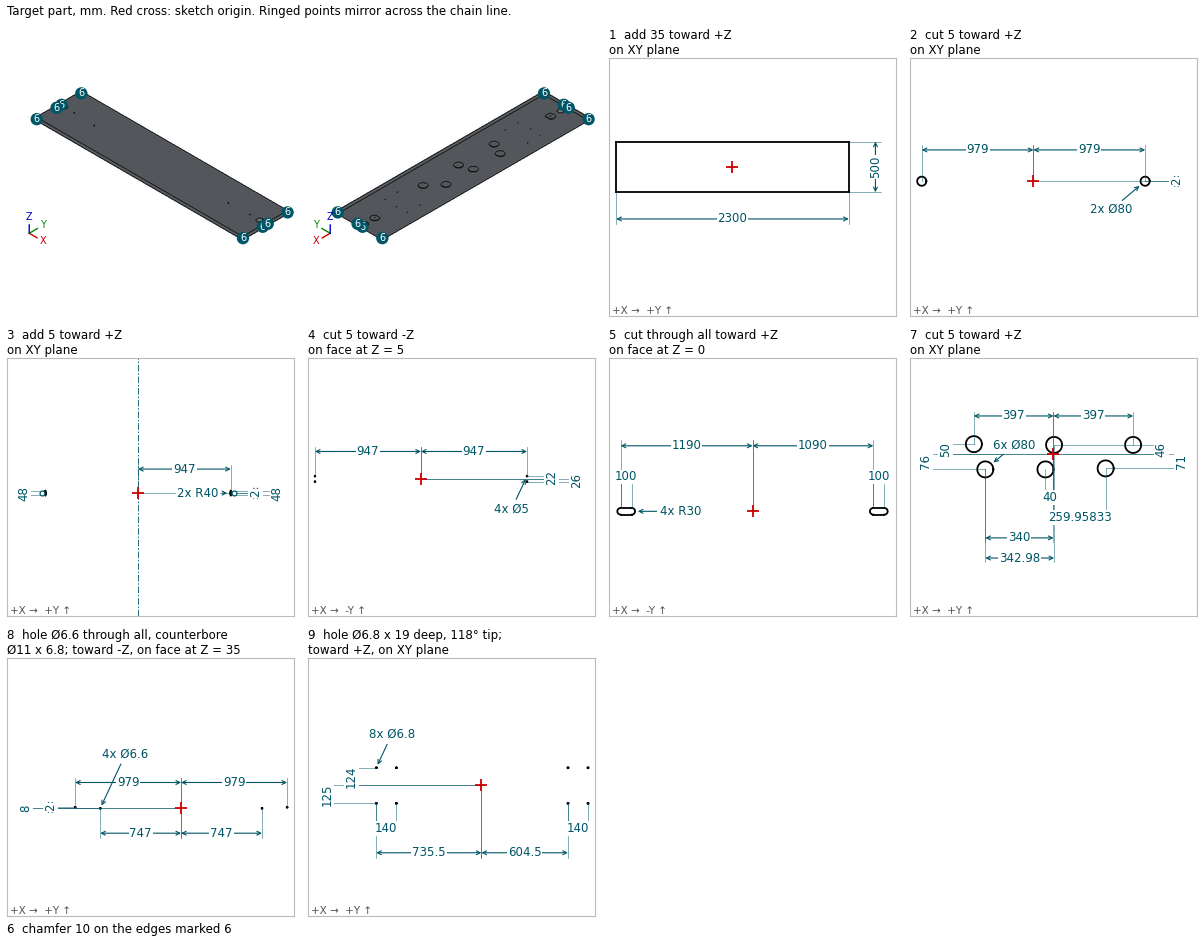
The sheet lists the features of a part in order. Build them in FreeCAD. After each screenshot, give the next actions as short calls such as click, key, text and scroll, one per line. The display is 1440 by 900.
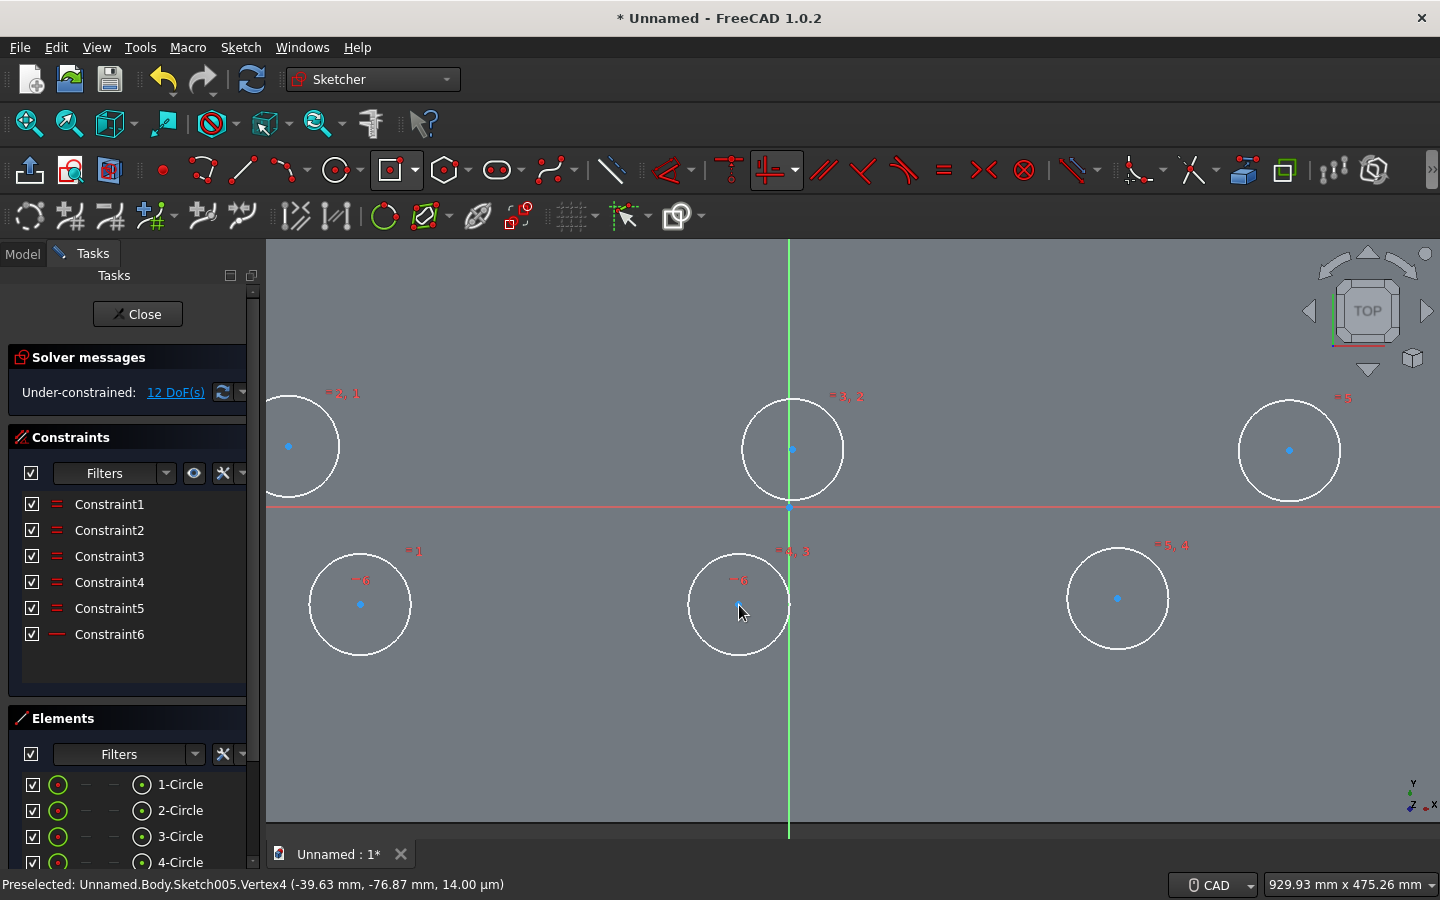
click(793, 450)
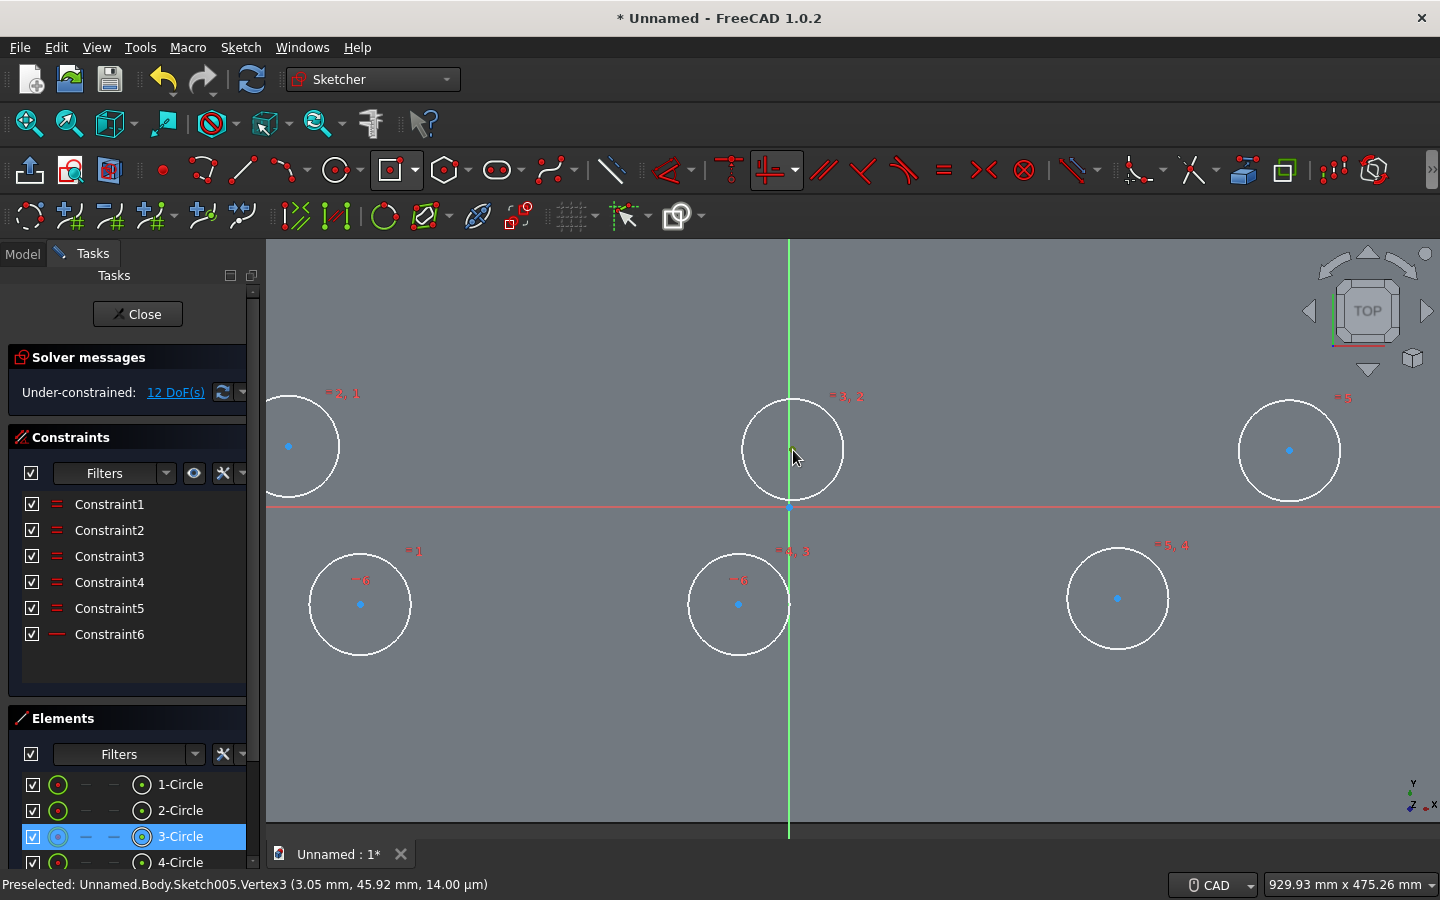
scroll(775, 570, down, 2)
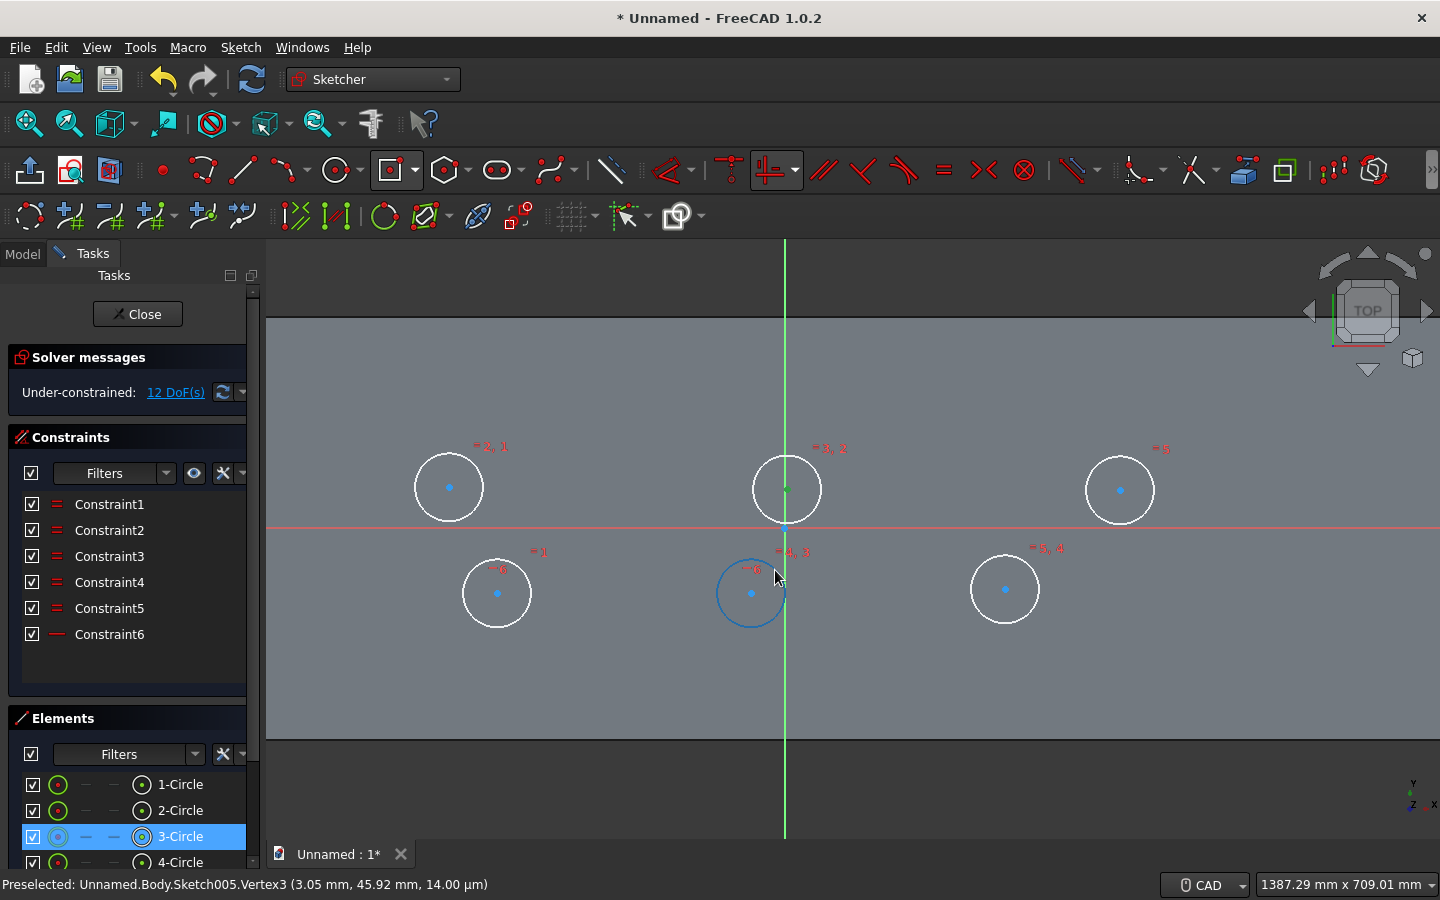
click(1120, 490)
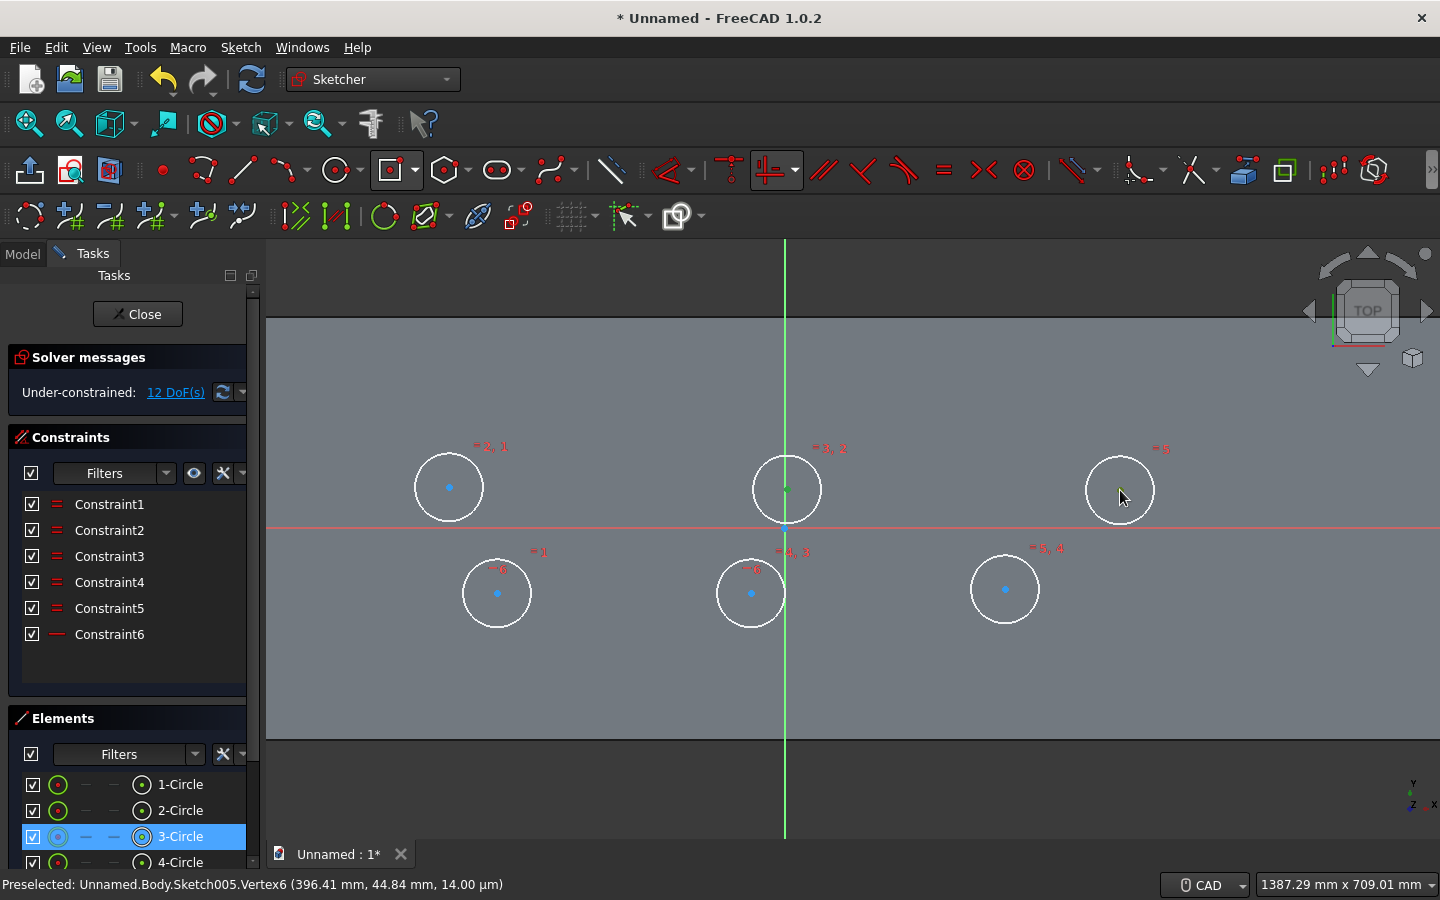
key(h)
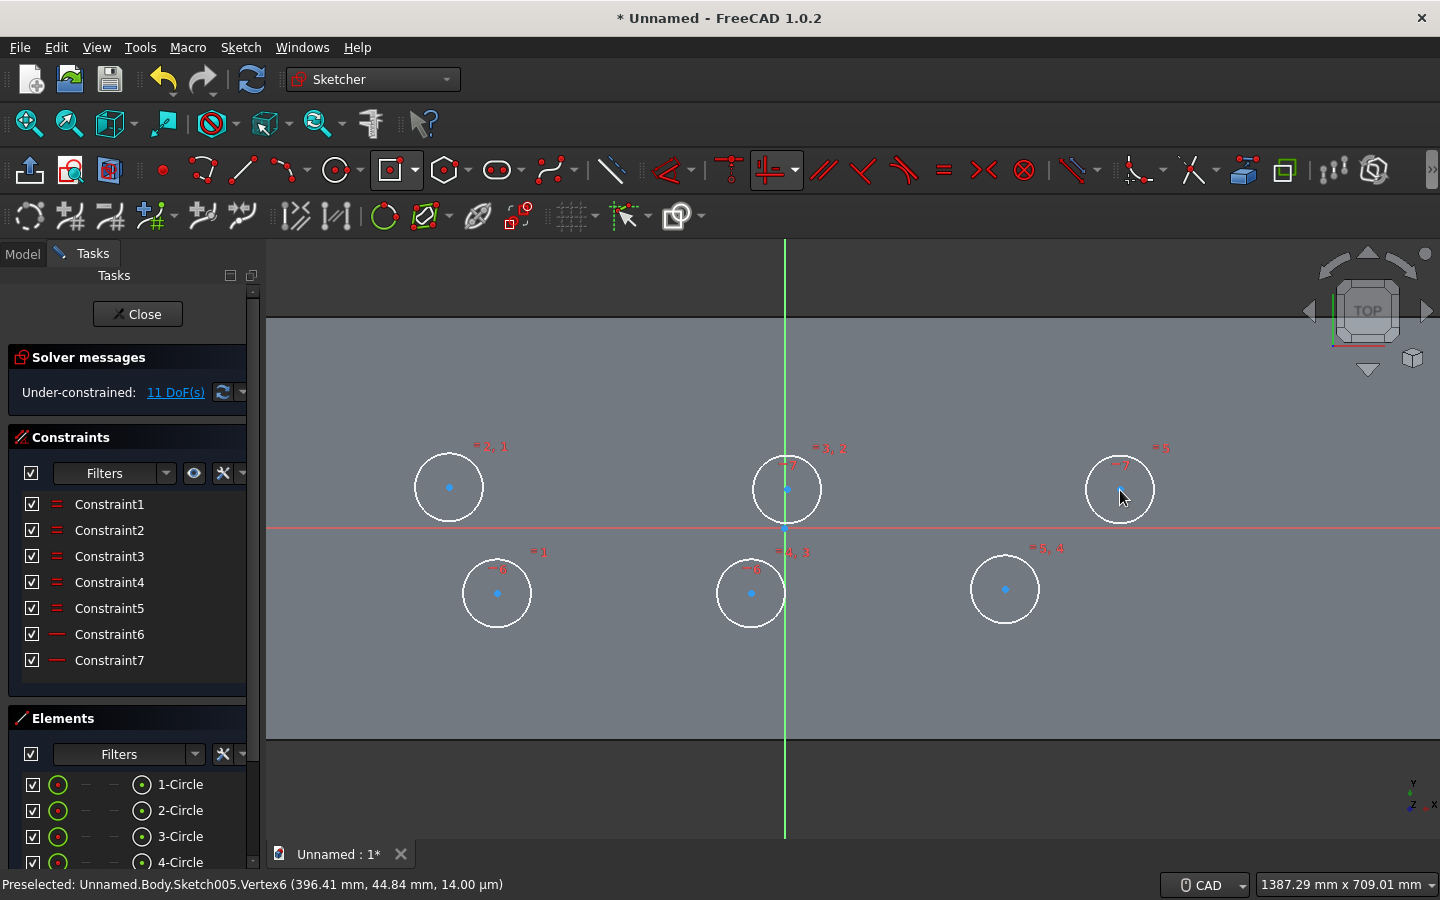
click(666, 170)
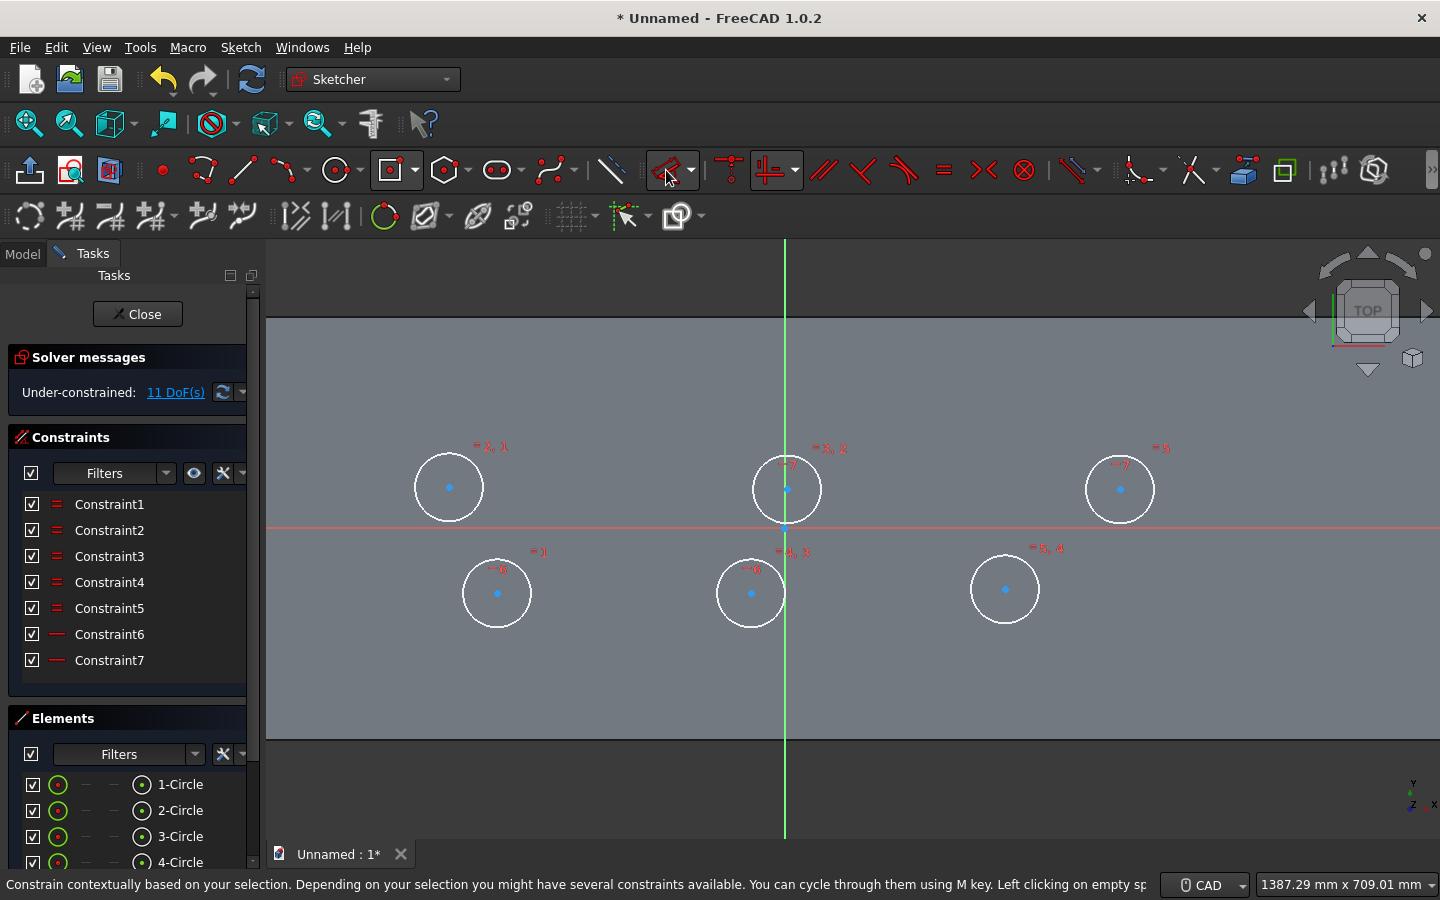
click(521, 569)
click(543, 546)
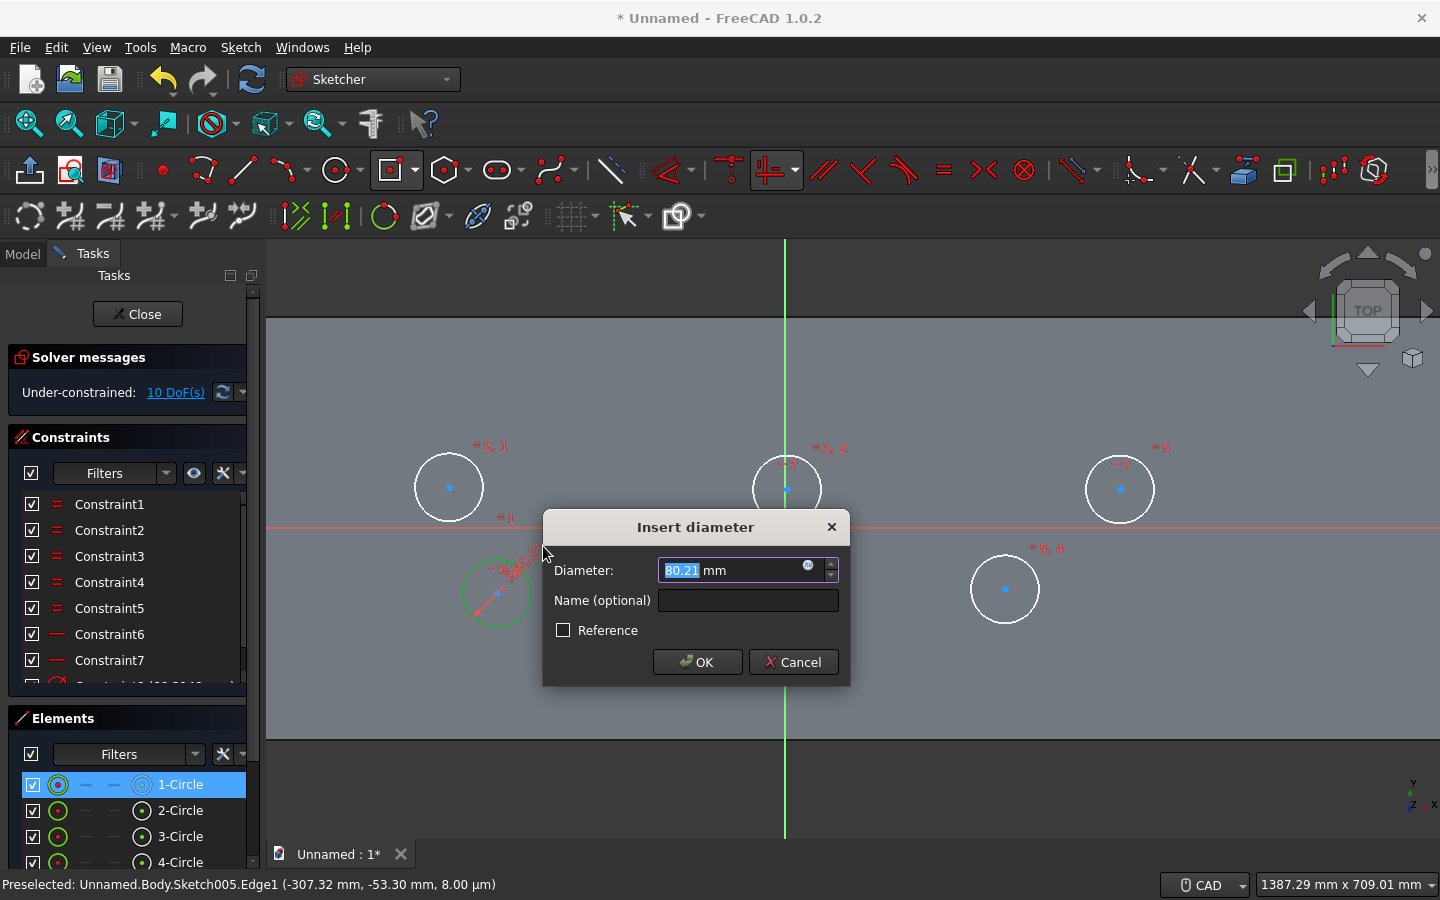
text(80)
key(Return)